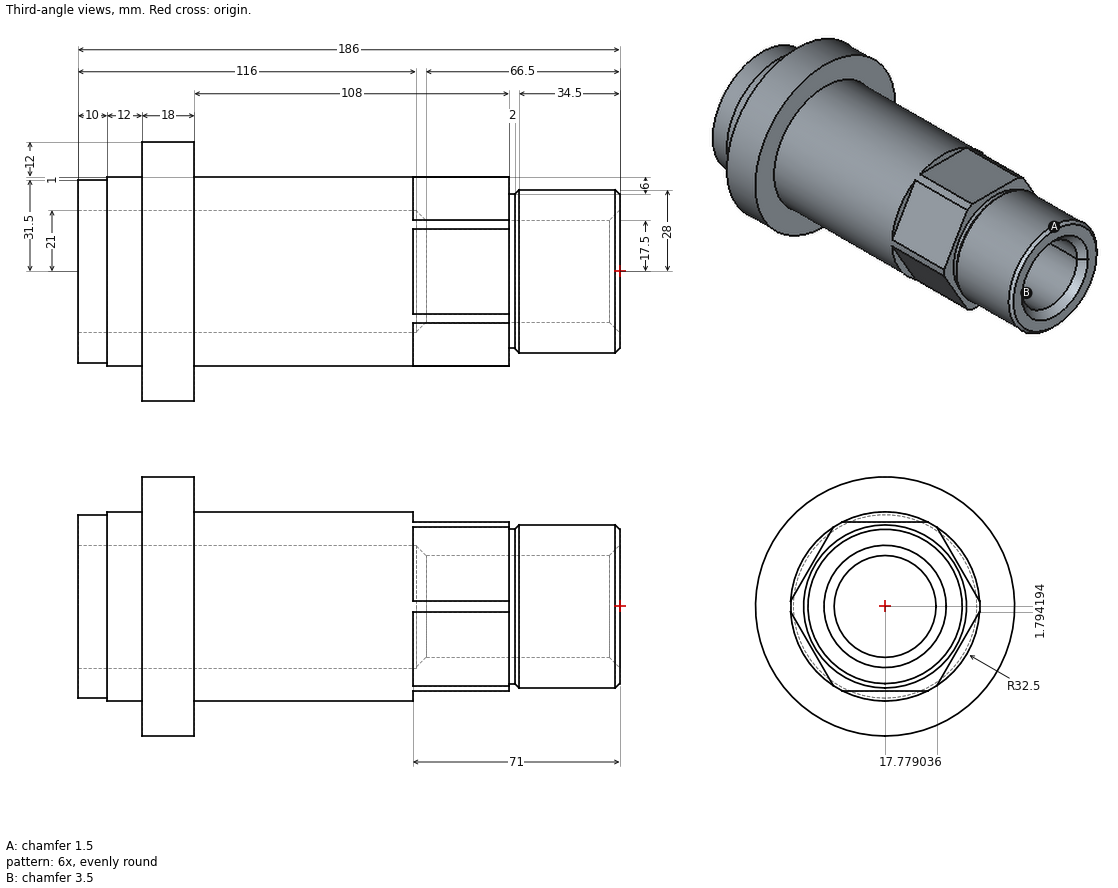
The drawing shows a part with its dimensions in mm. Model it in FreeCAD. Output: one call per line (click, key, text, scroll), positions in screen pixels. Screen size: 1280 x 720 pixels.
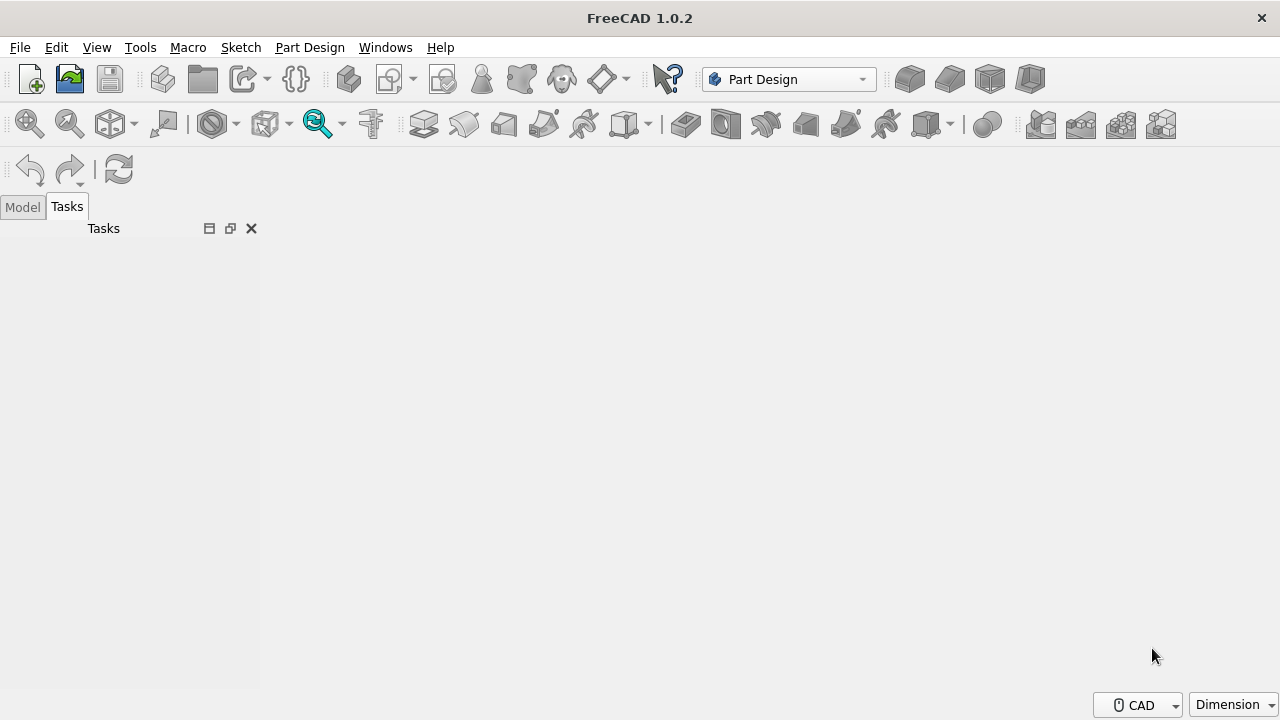
click(30, 80)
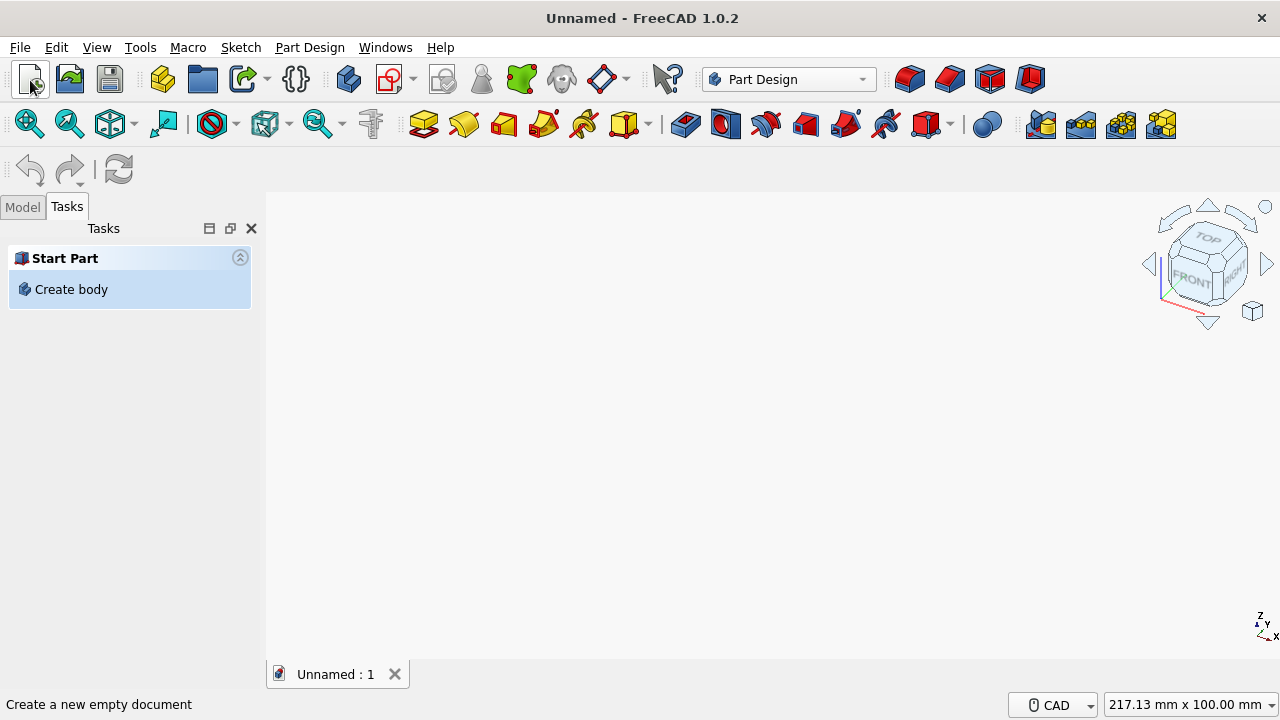
click(390, 80)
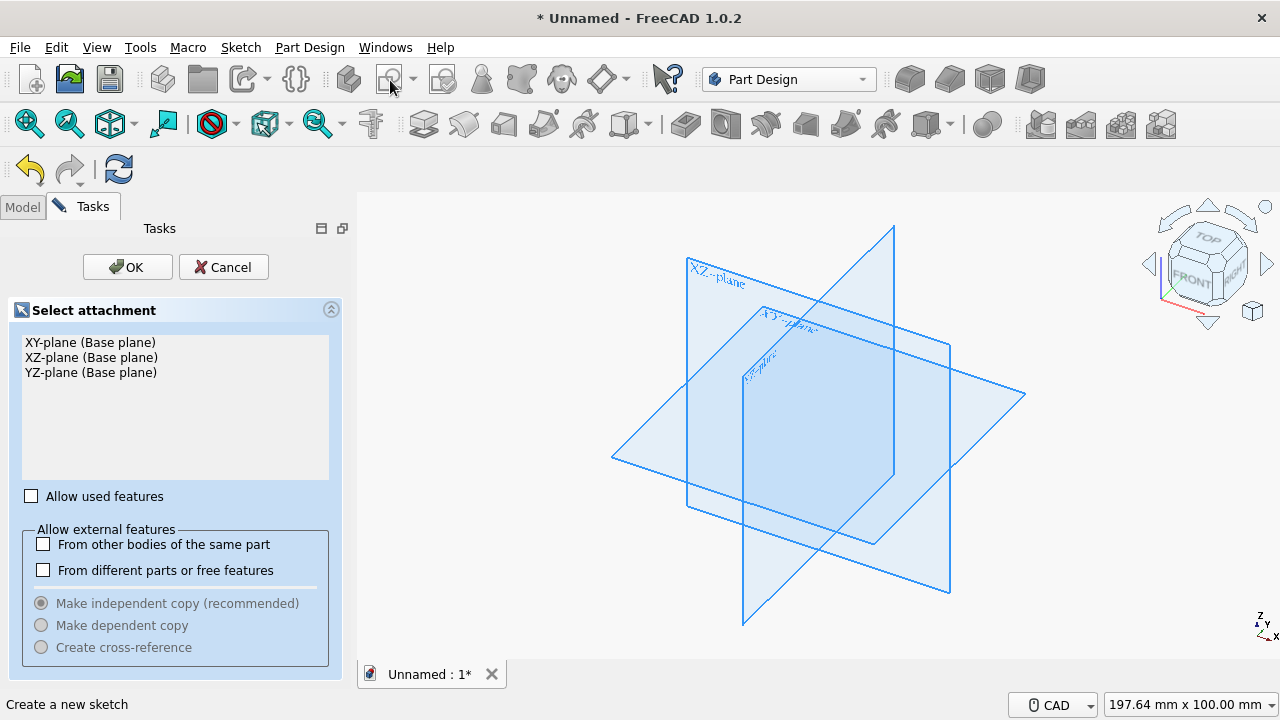
click(82, 342)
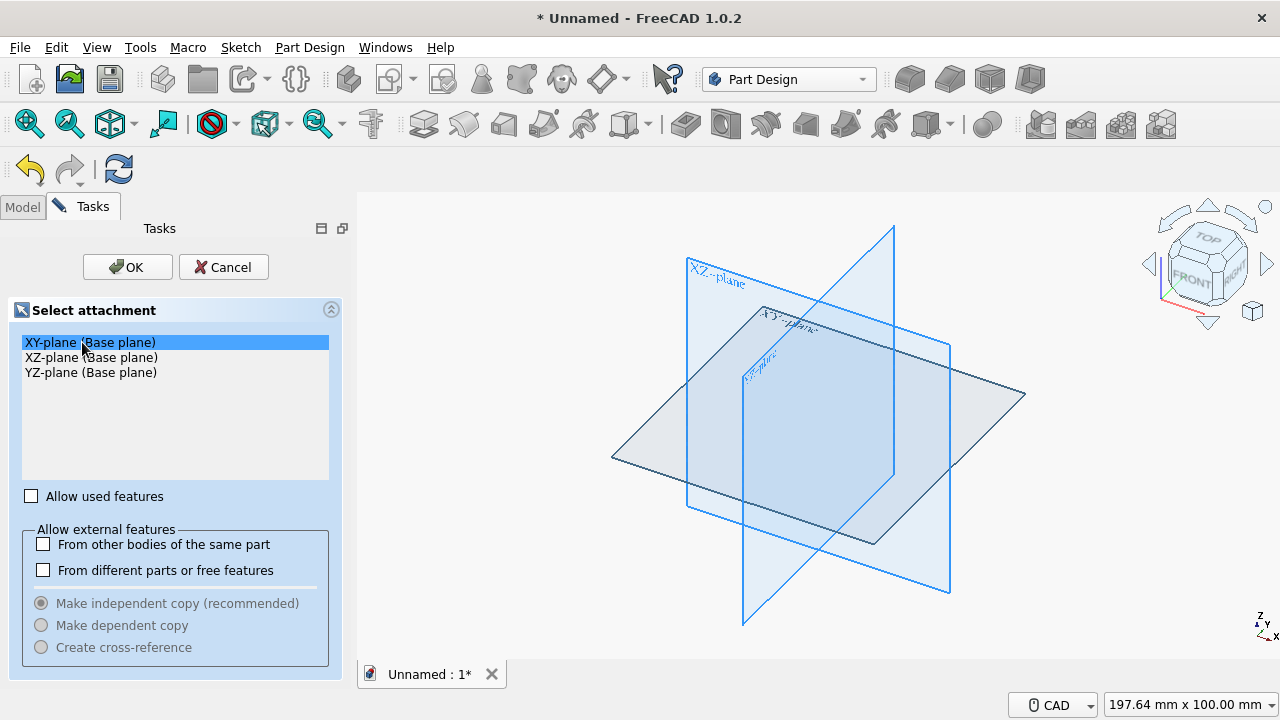
click(128, 267)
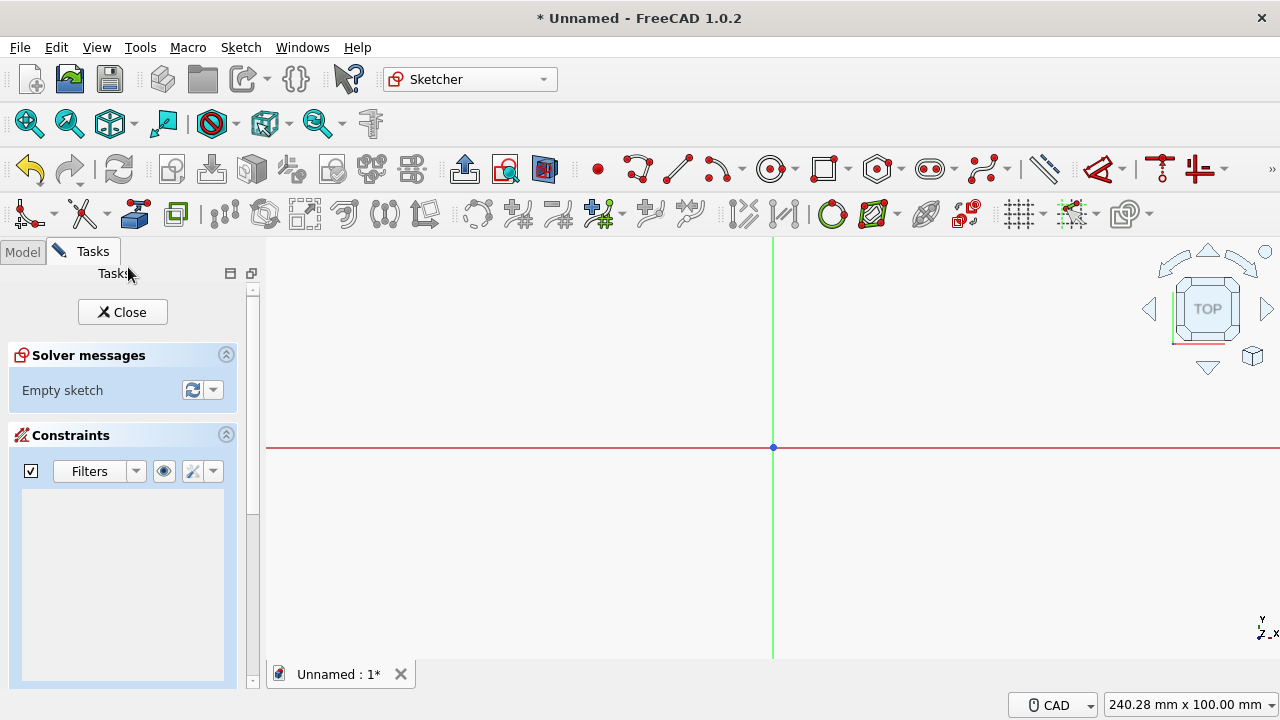
scroll(1115, 631, down, 2)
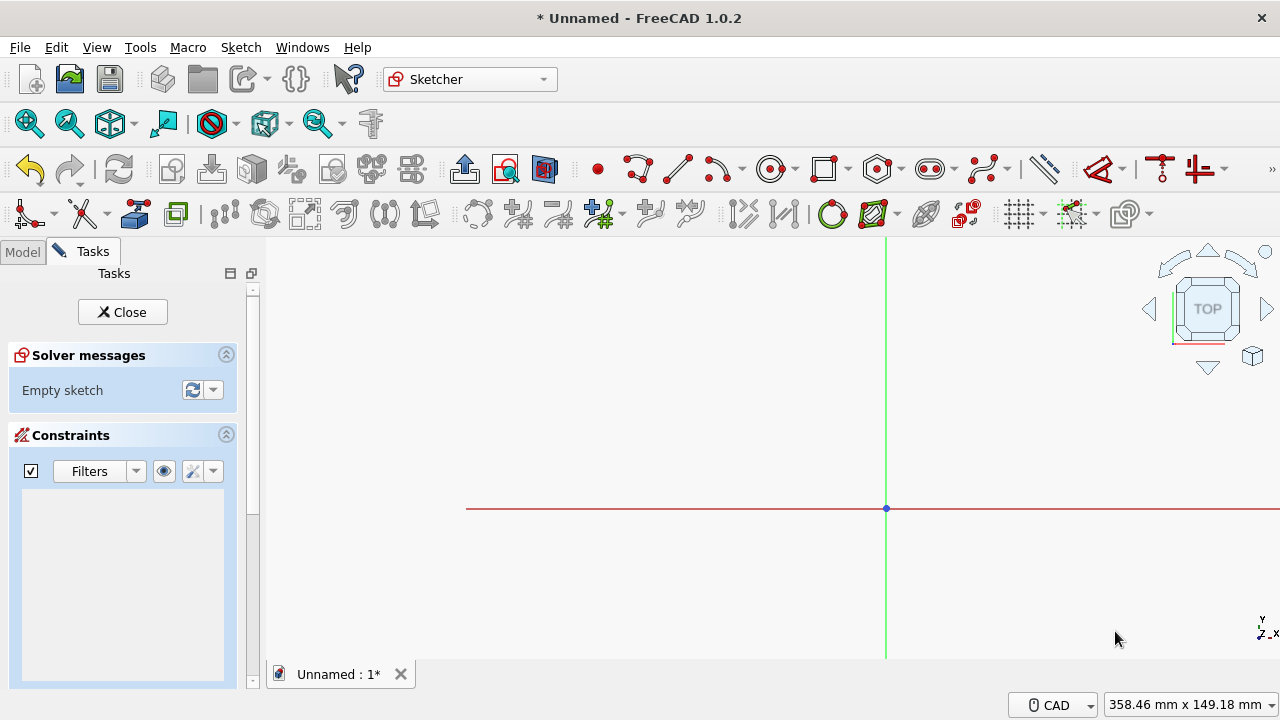
click(638, 170)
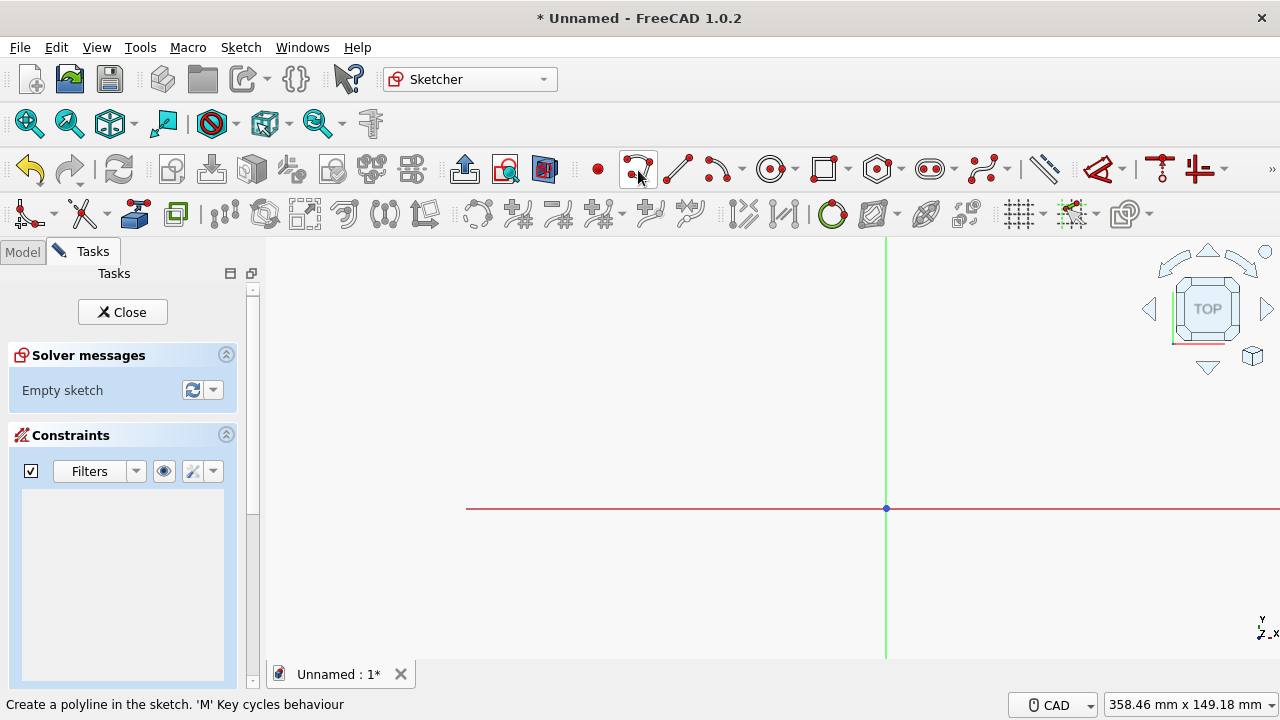
click(886, 509)
click(877, 429)
click(788, 429)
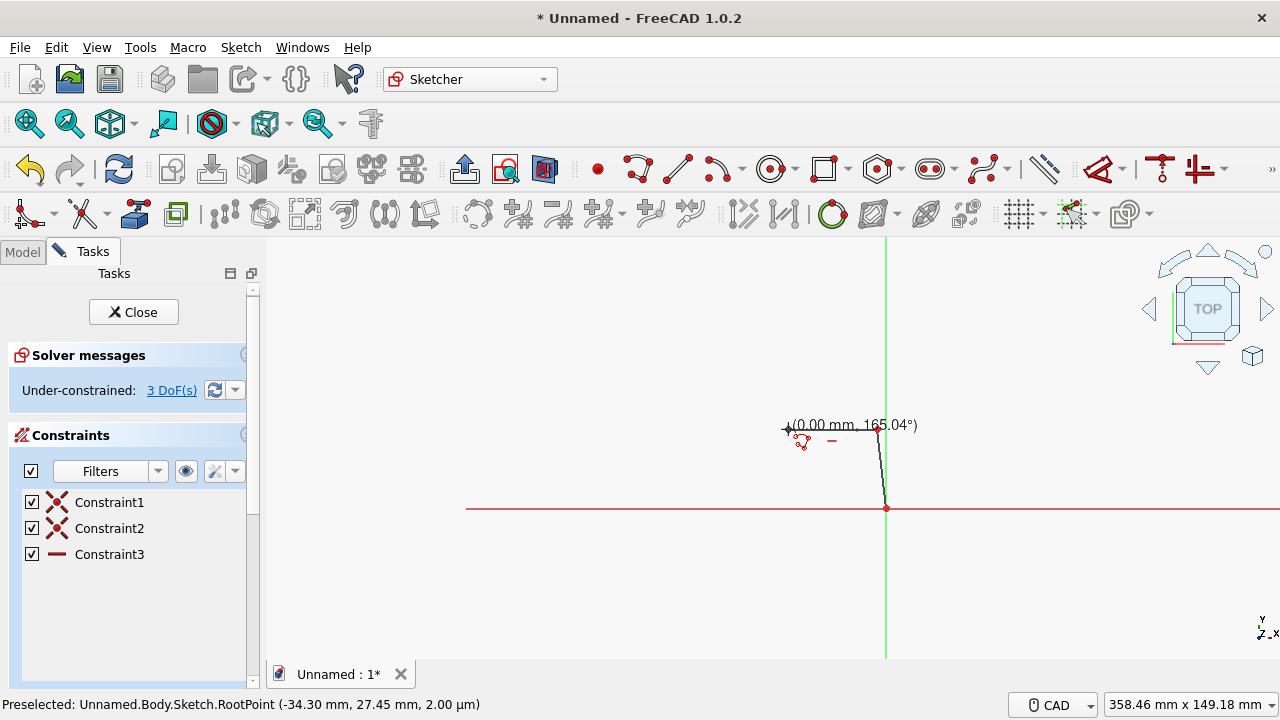
scroll(784, 434, up, 5)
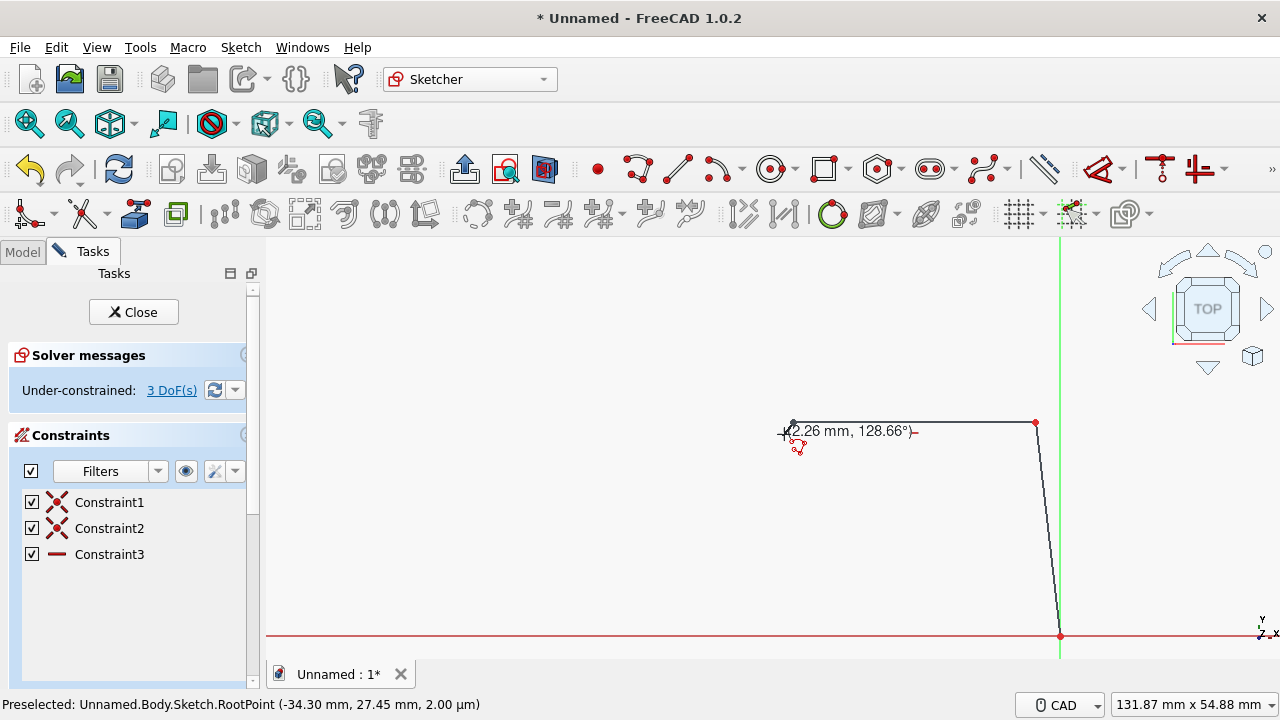
click(784, 432)
click(768, 432)
click(768, 386)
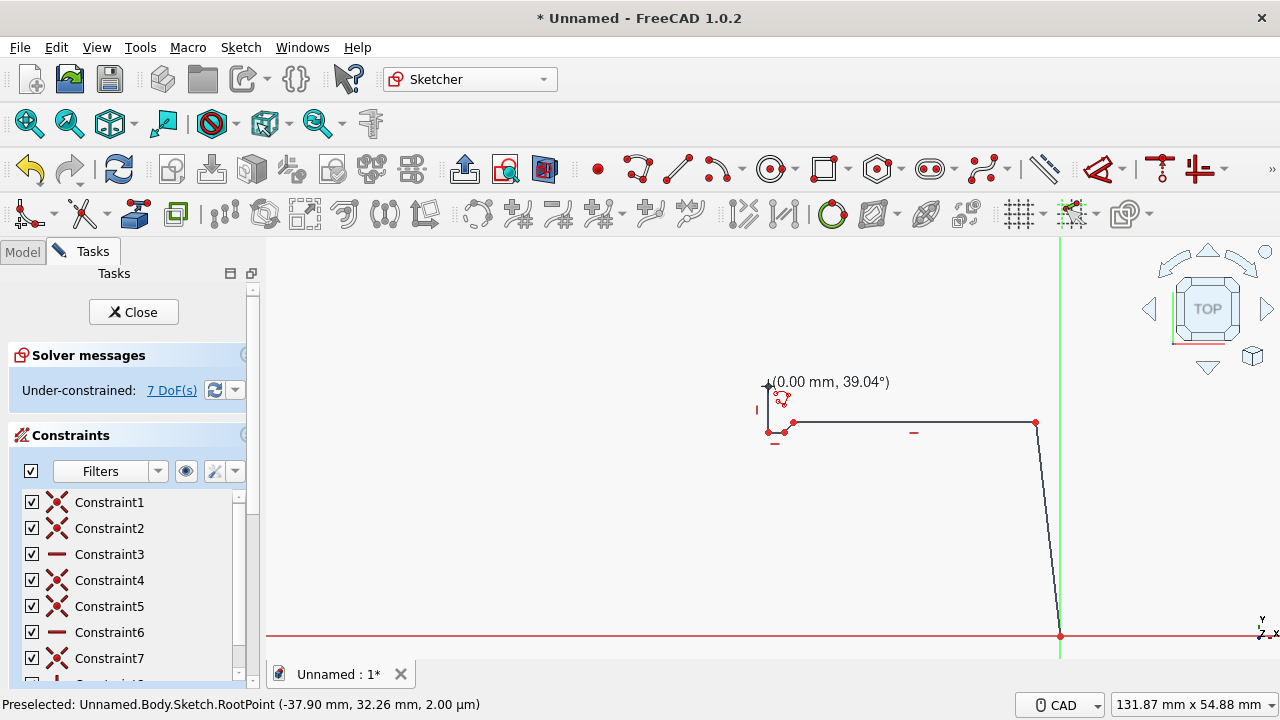
scroll(914, 438, down, 5)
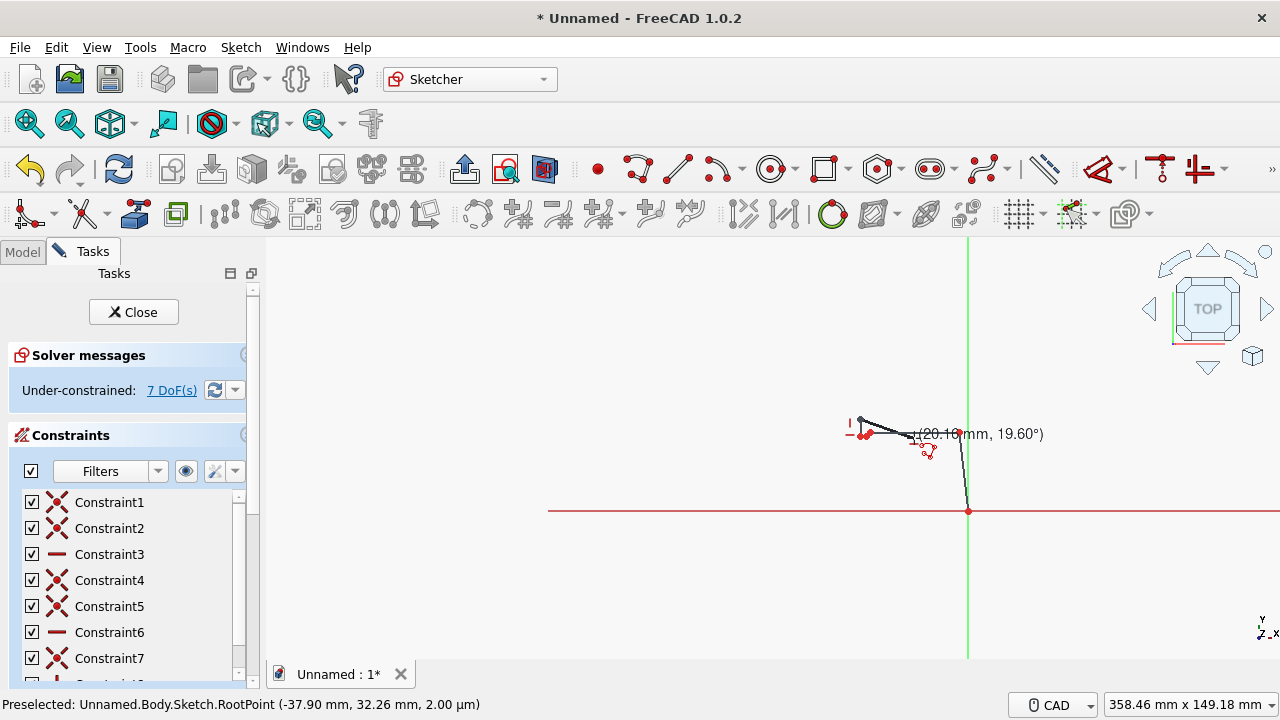
click(555, 419)
click(555, 385)
click(504, 385)
click(504, 419)
click(470, 419)